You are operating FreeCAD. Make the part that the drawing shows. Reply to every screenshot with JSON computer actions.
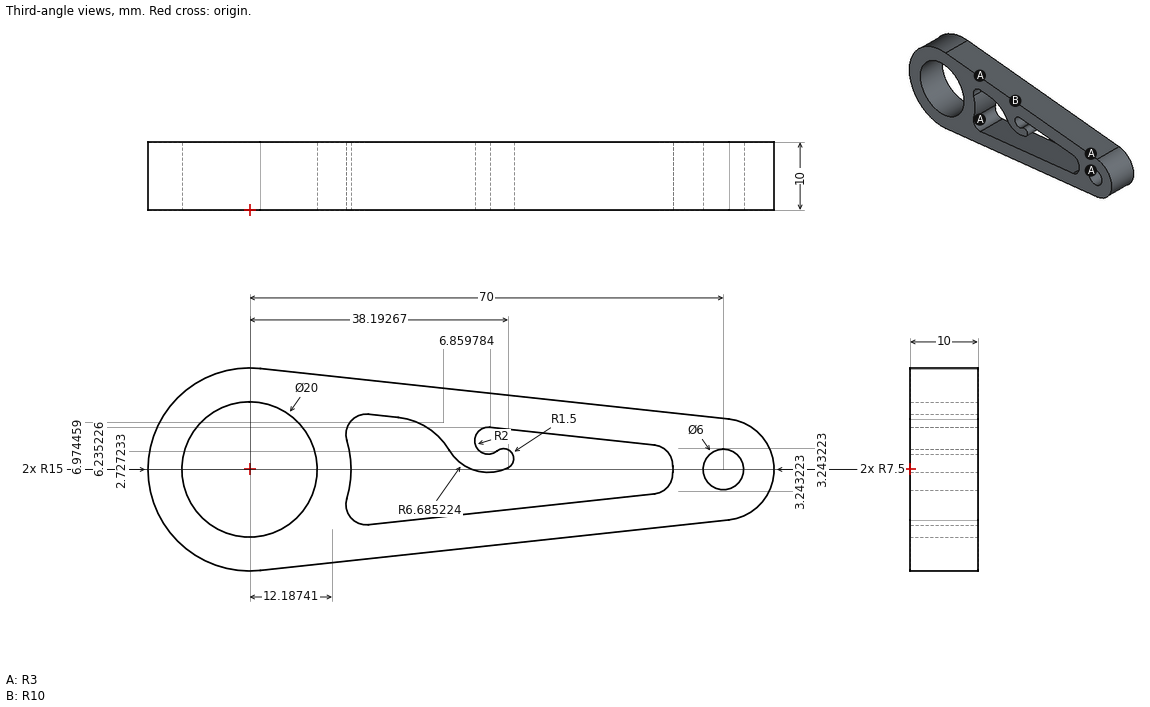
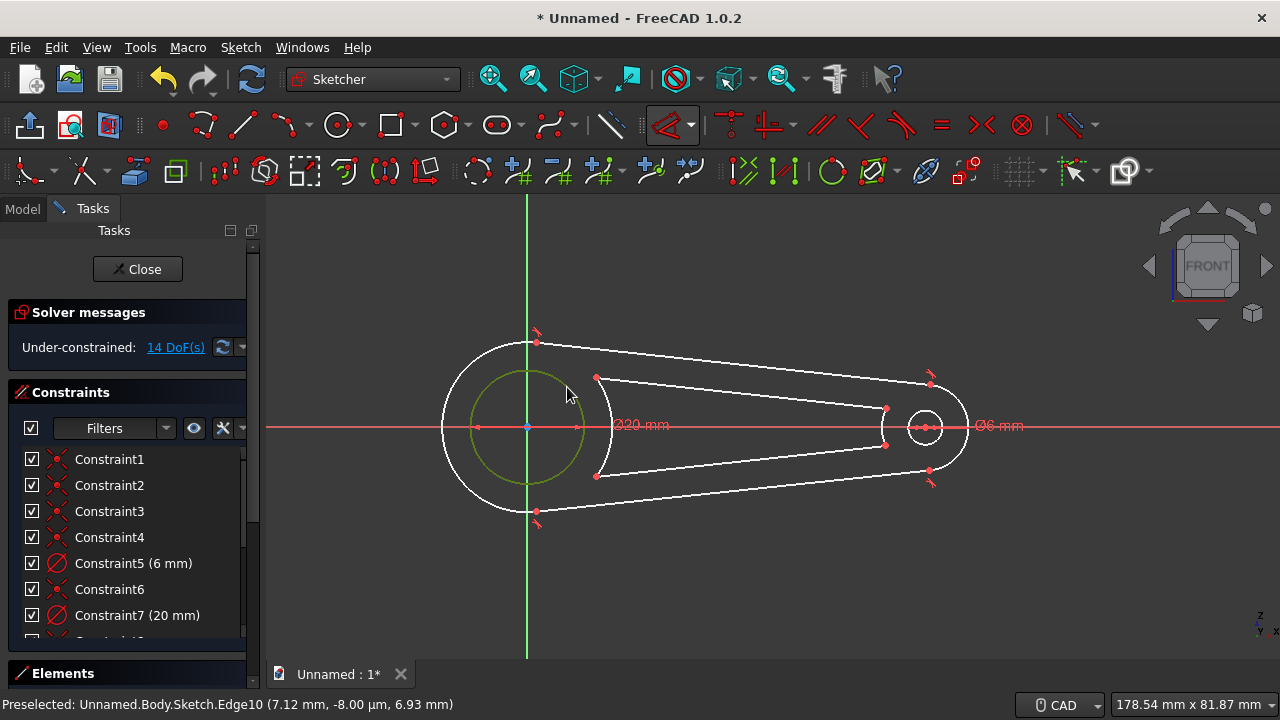
{"action": "left_click", "coordinate": [609, 448]}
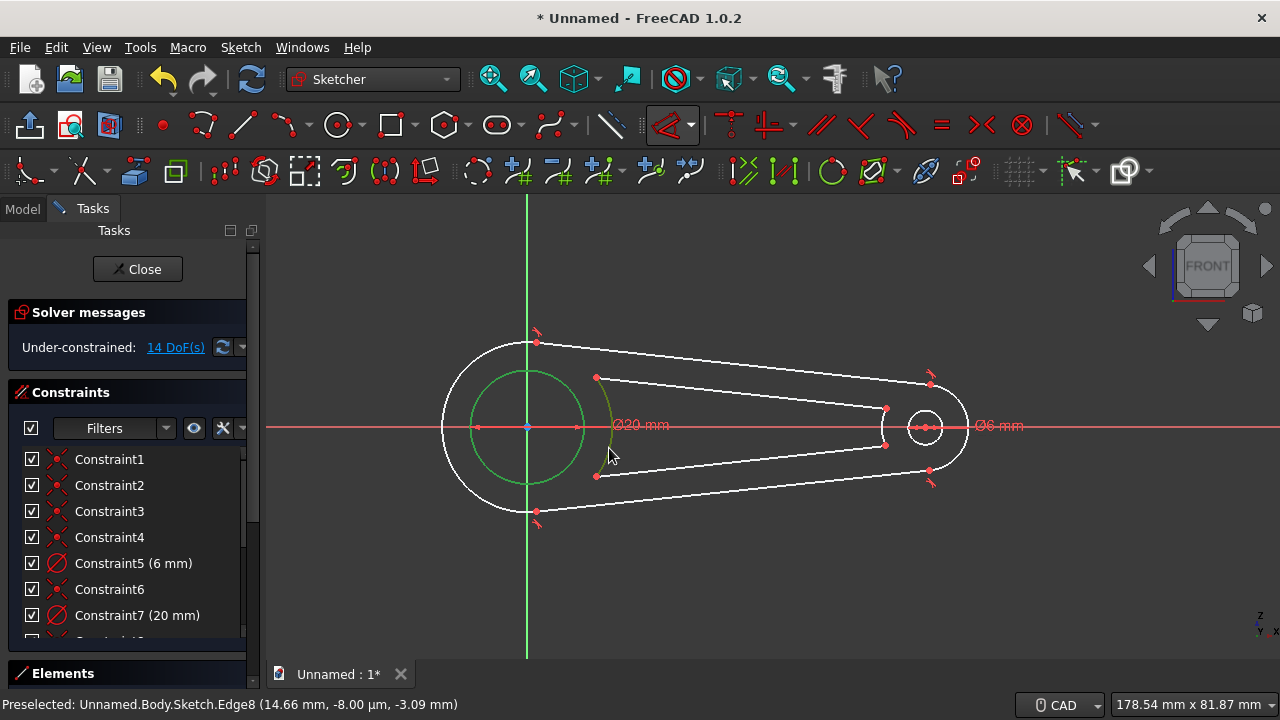
{"action": "left_click", "coordinate": [730, 126]}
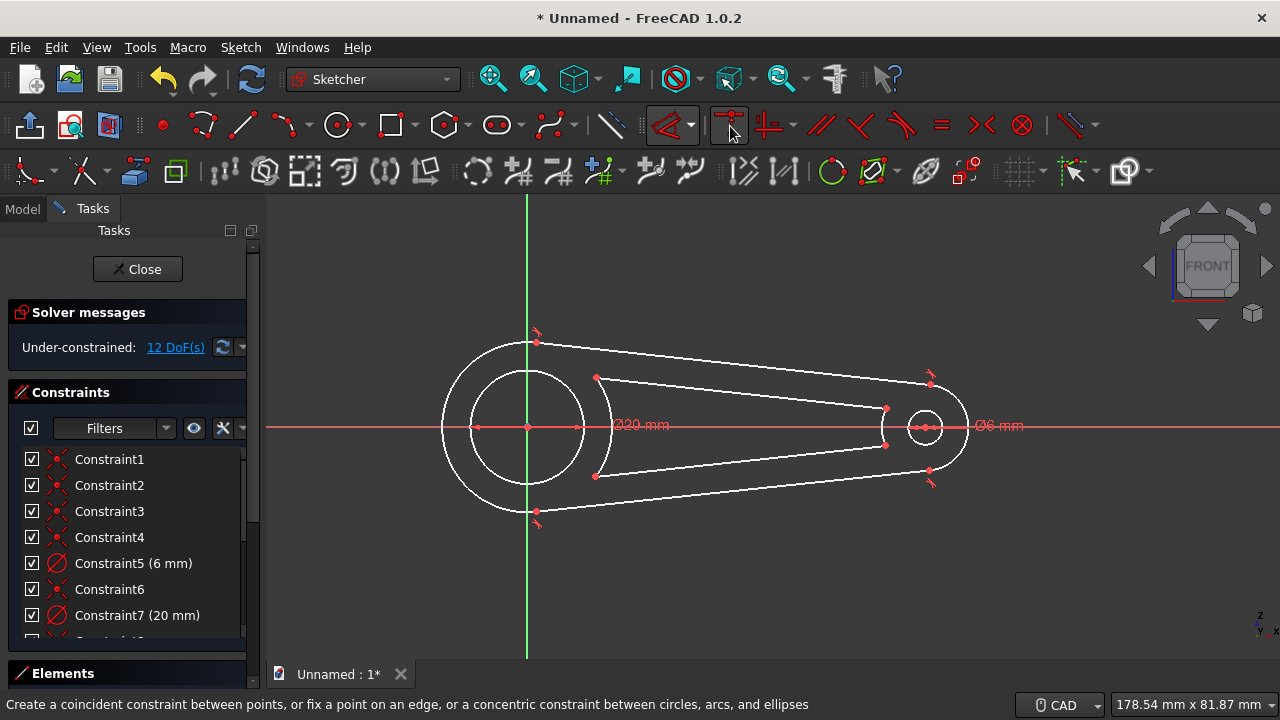
{"action": "scroll", "coordinate": [527, 427], "scroll_direction": "up", "scroll_amount": 5}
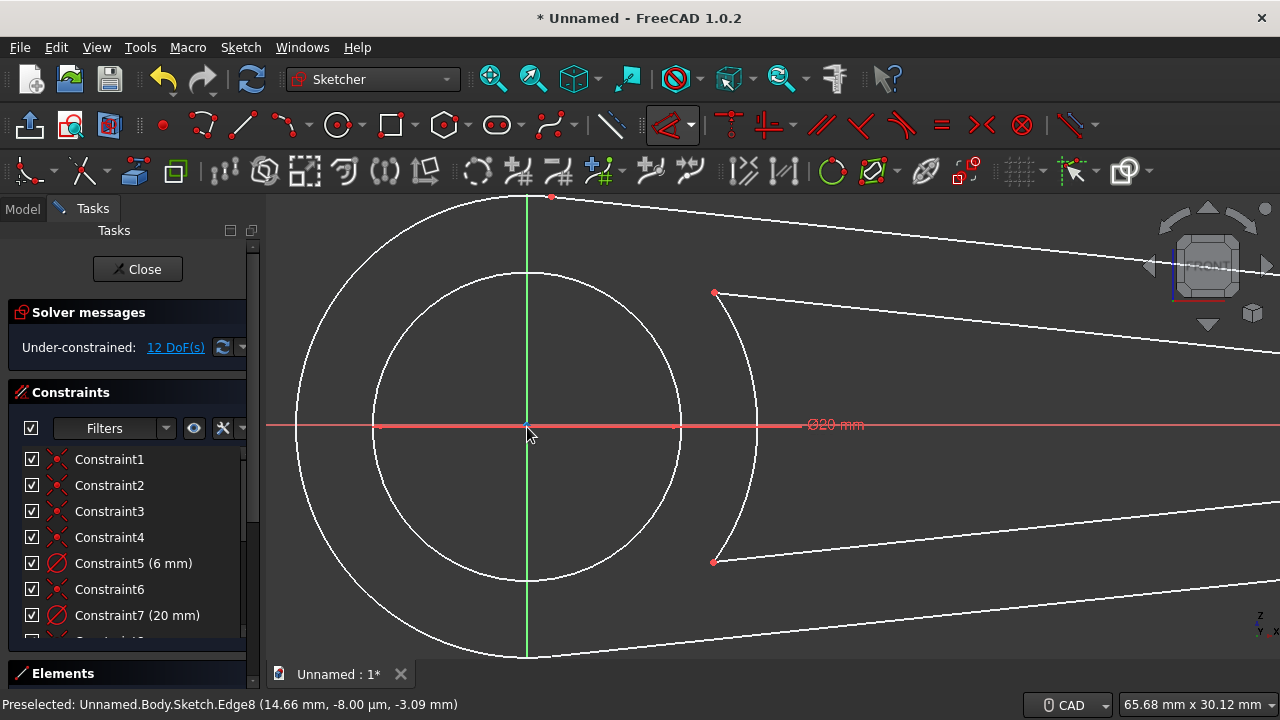
{"action": "left_click_drag", "start_coordinate": [517, 415], "coordinate": [537, 437]}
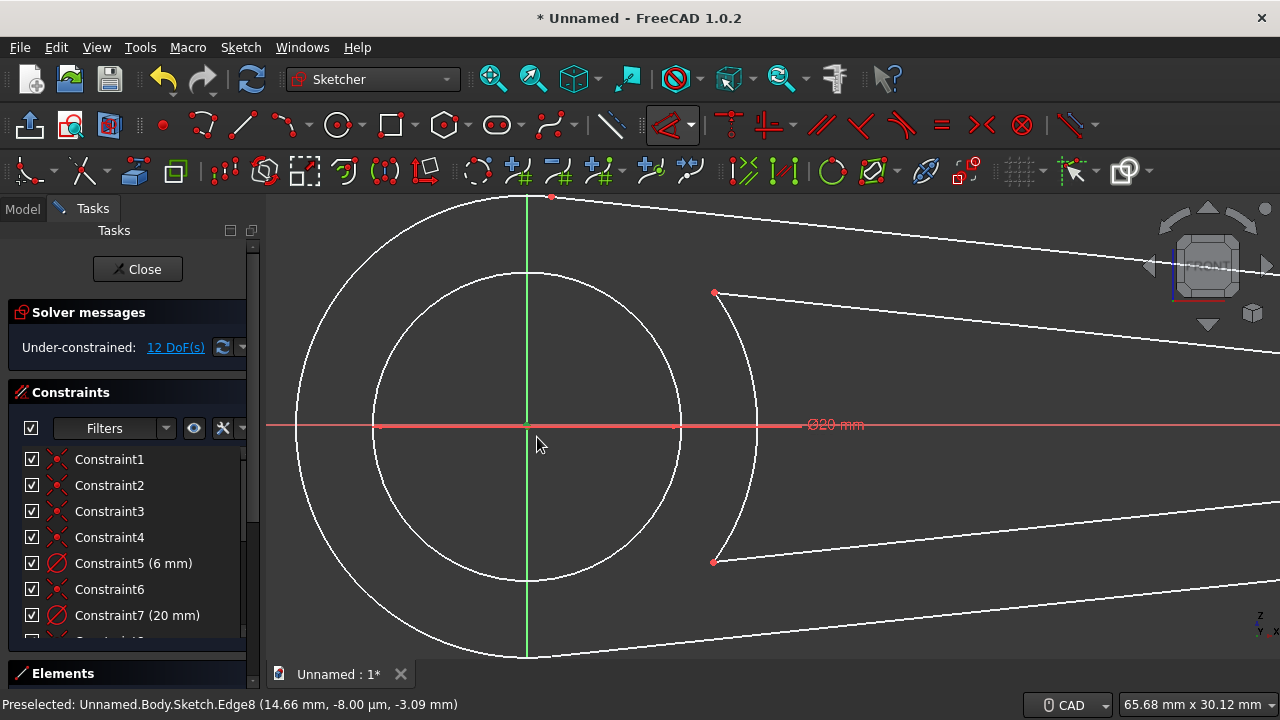
{"action": "left_click", "coordinate": [730, 126]}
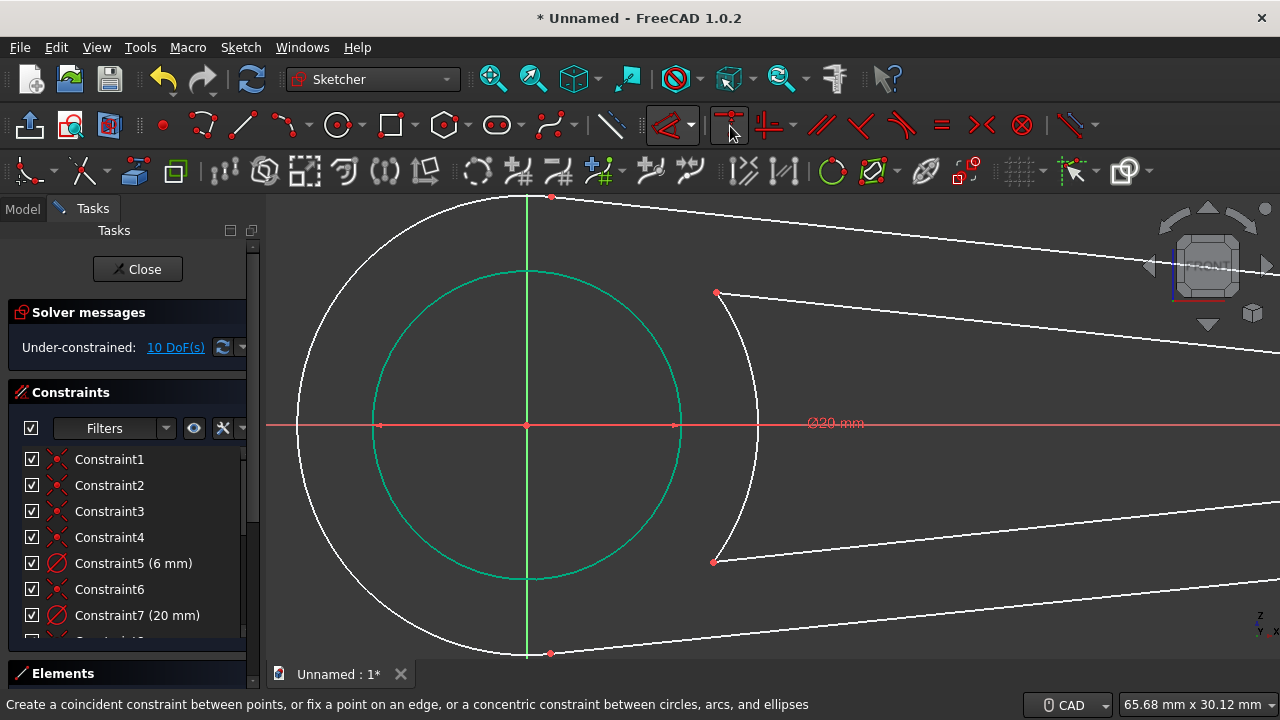
{"action": "scroll", "coordinate": [527, 427], "scroll_direction": "down", "scroll_amount": 5}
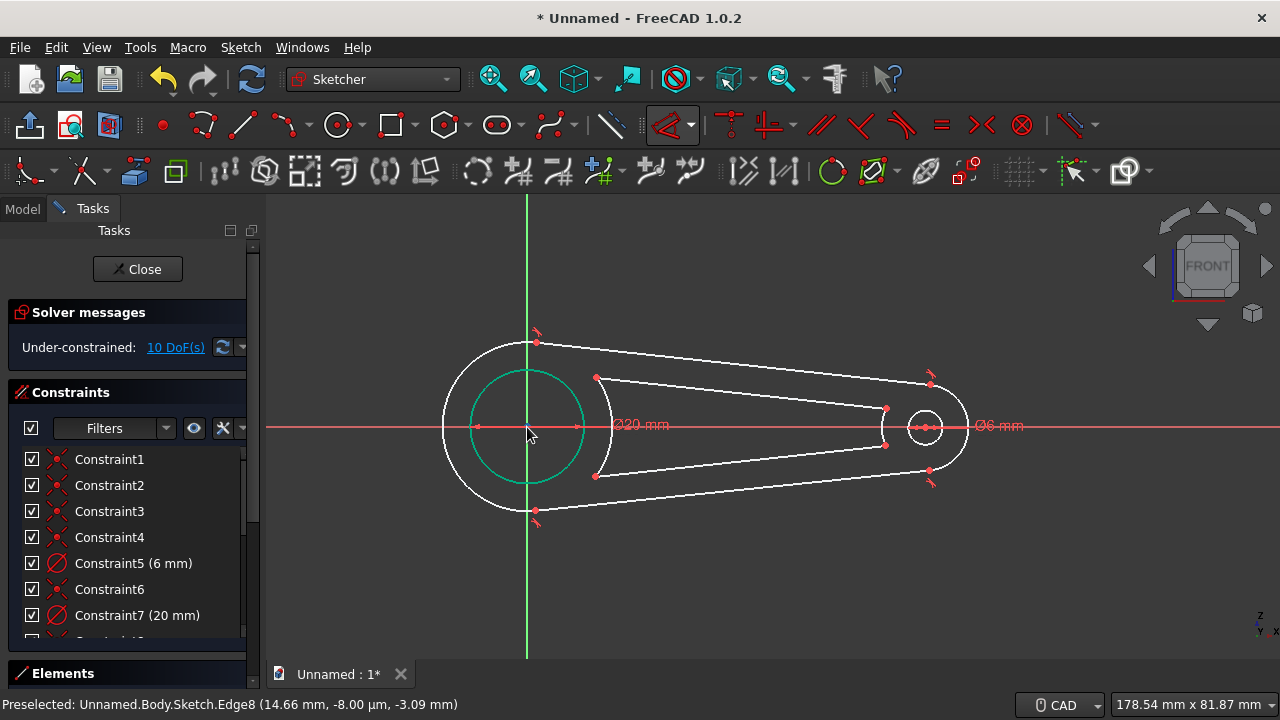
{"action": "left_click", "coordinate": [961, 452]}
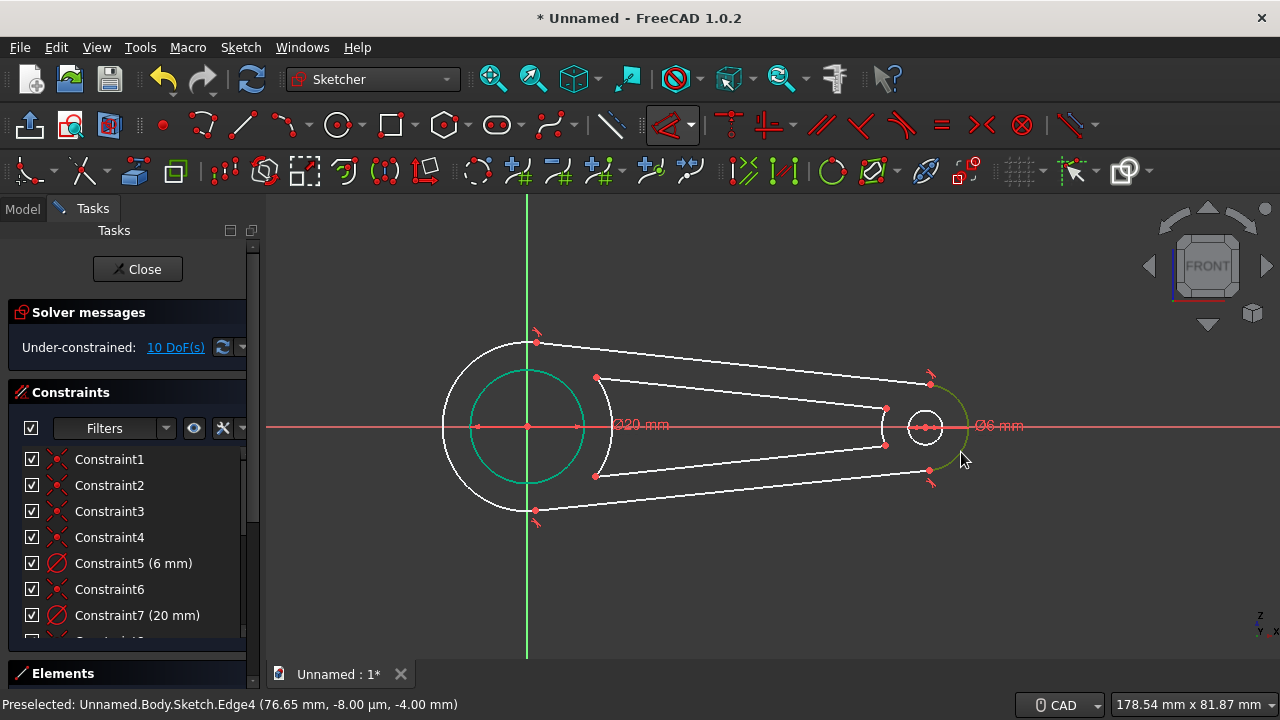
{"action": "left_click", "coordinate": [882, 427]}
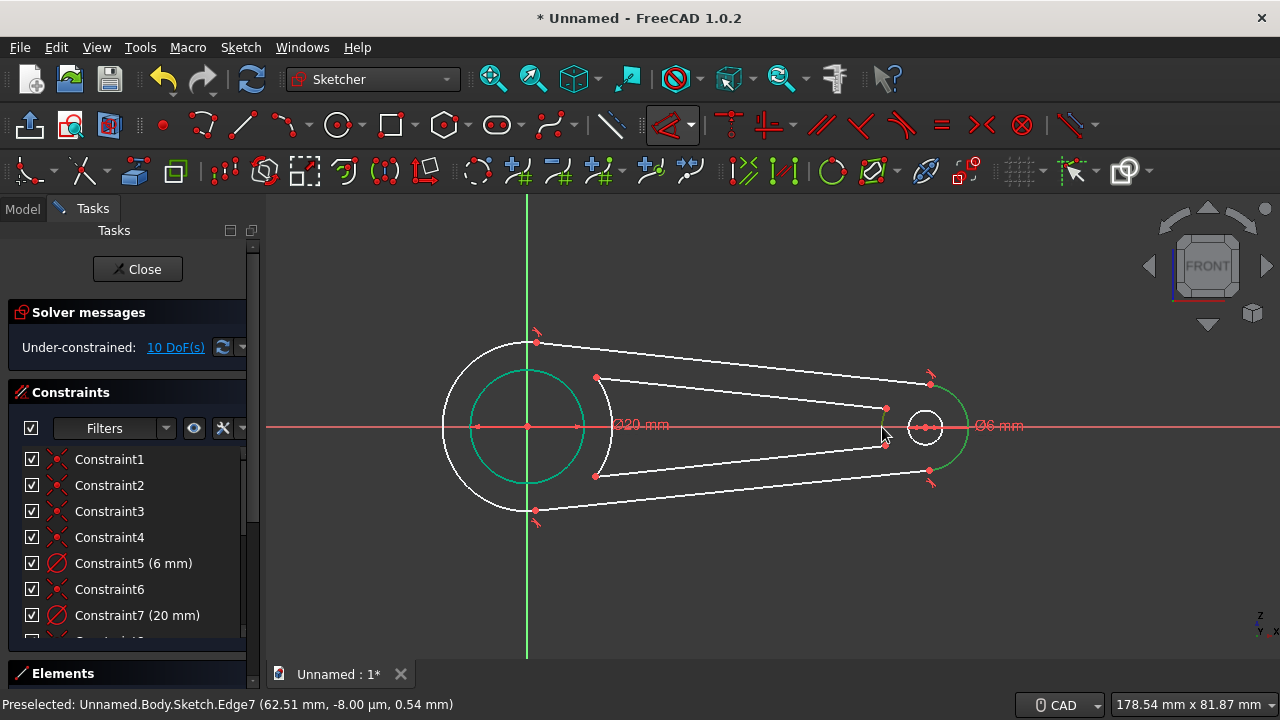
{"action": "left_click", "coordinate": [942, 126]}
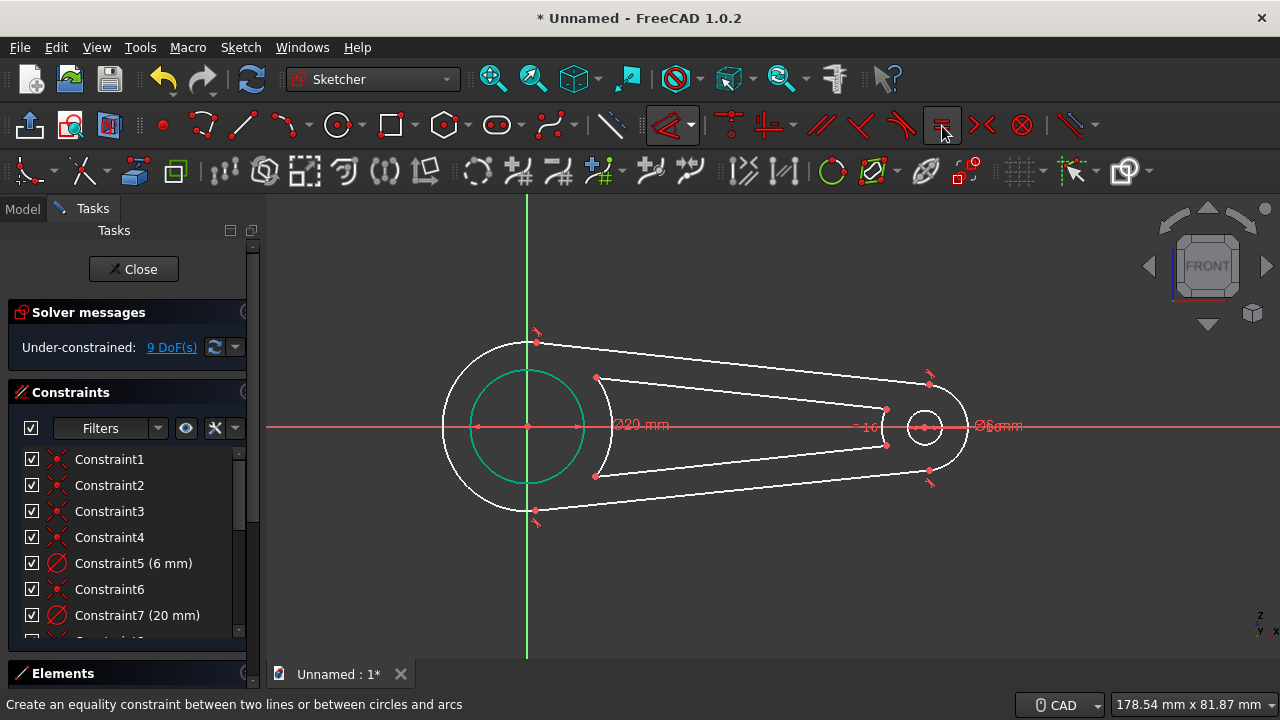
{"action": "left_click", "coordinate": [461, 374]}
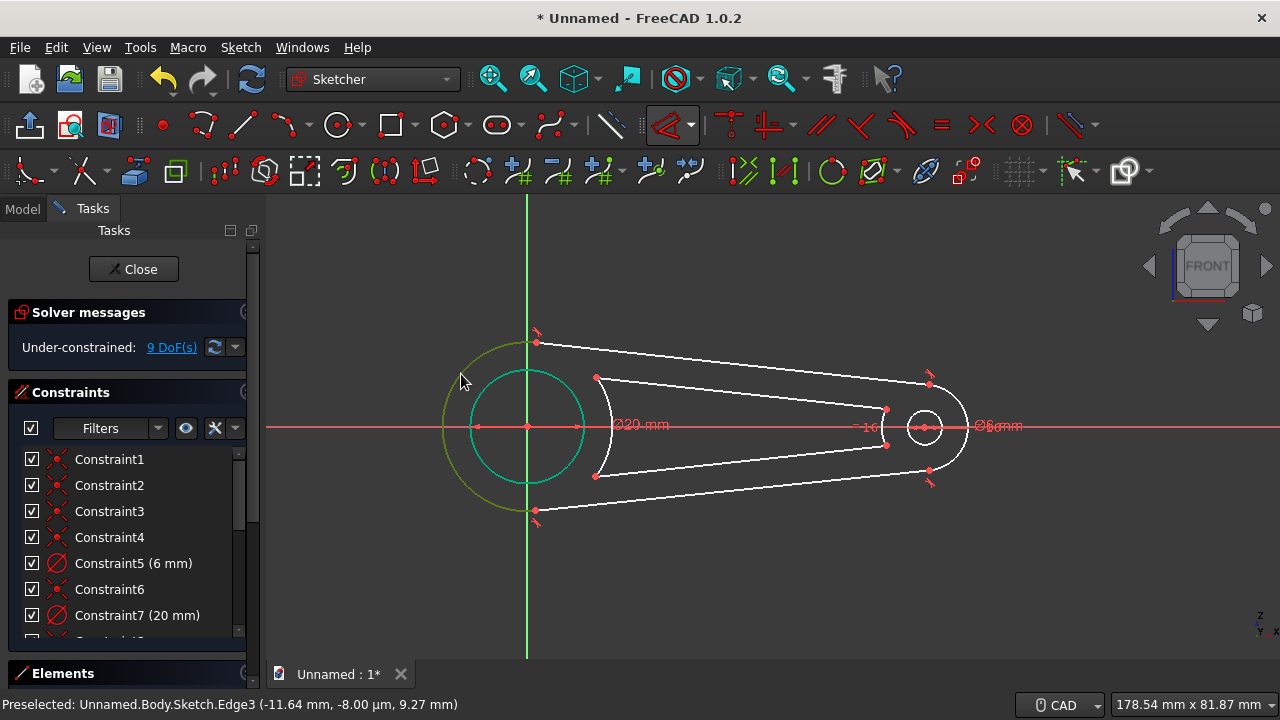
{"action": "left_click", "coordinate": [609, 449]}